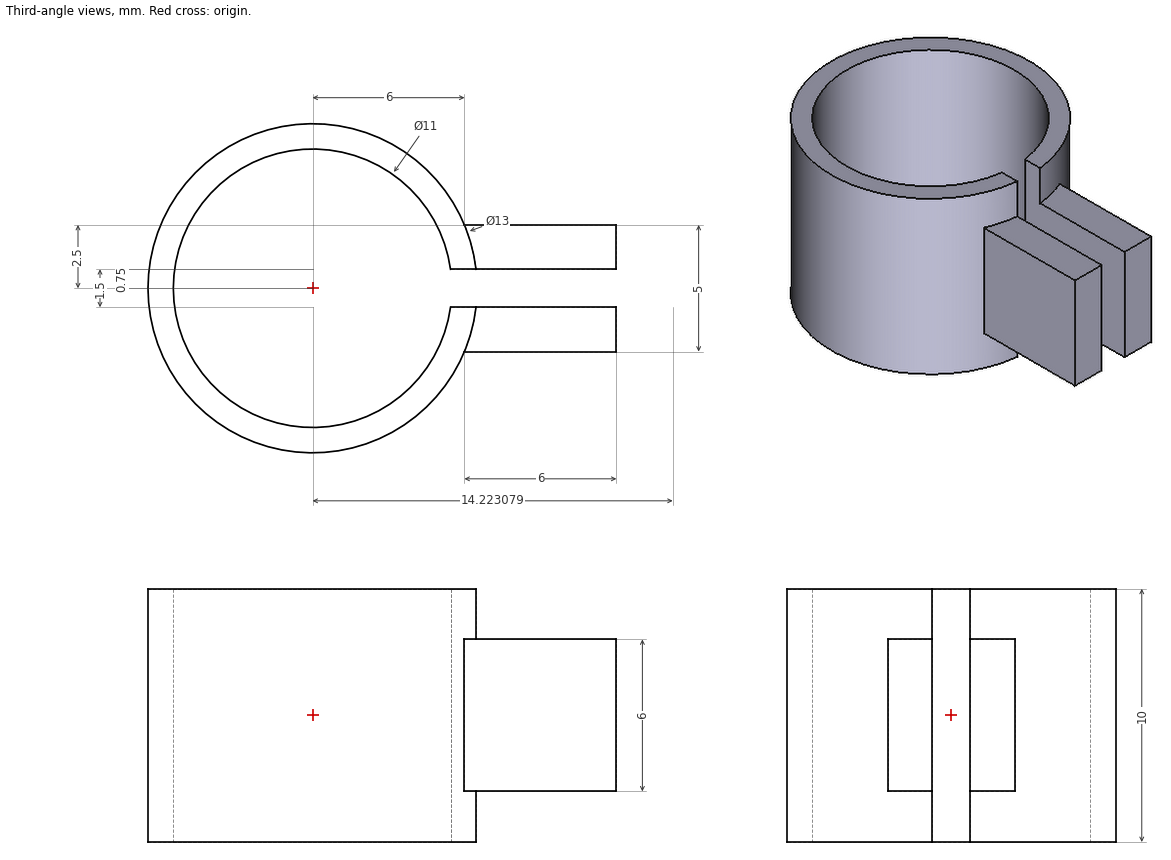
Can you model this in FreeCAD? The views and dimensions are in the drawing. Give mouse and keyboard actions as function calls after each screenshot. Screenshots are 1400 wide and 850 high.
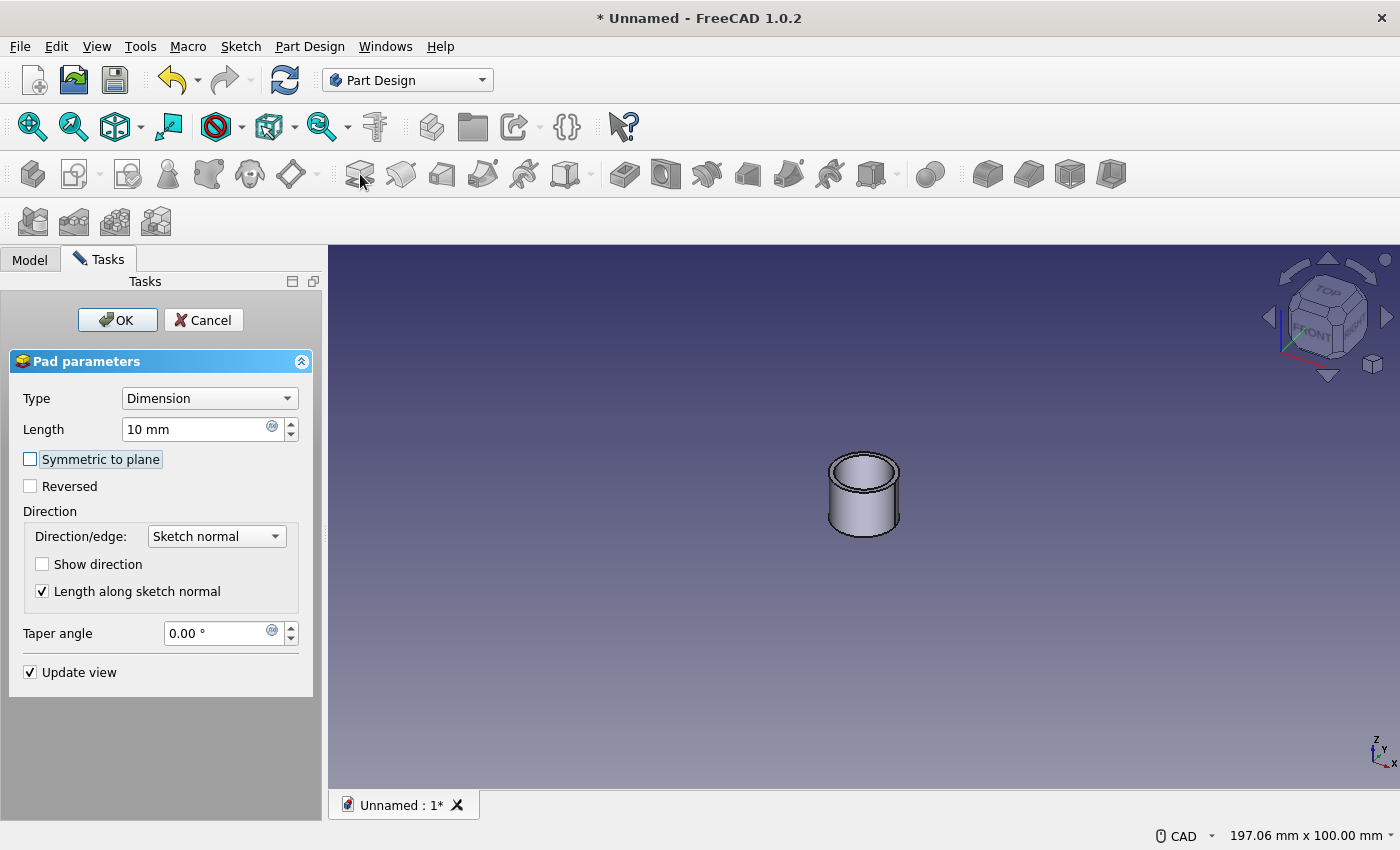
click(31, 459)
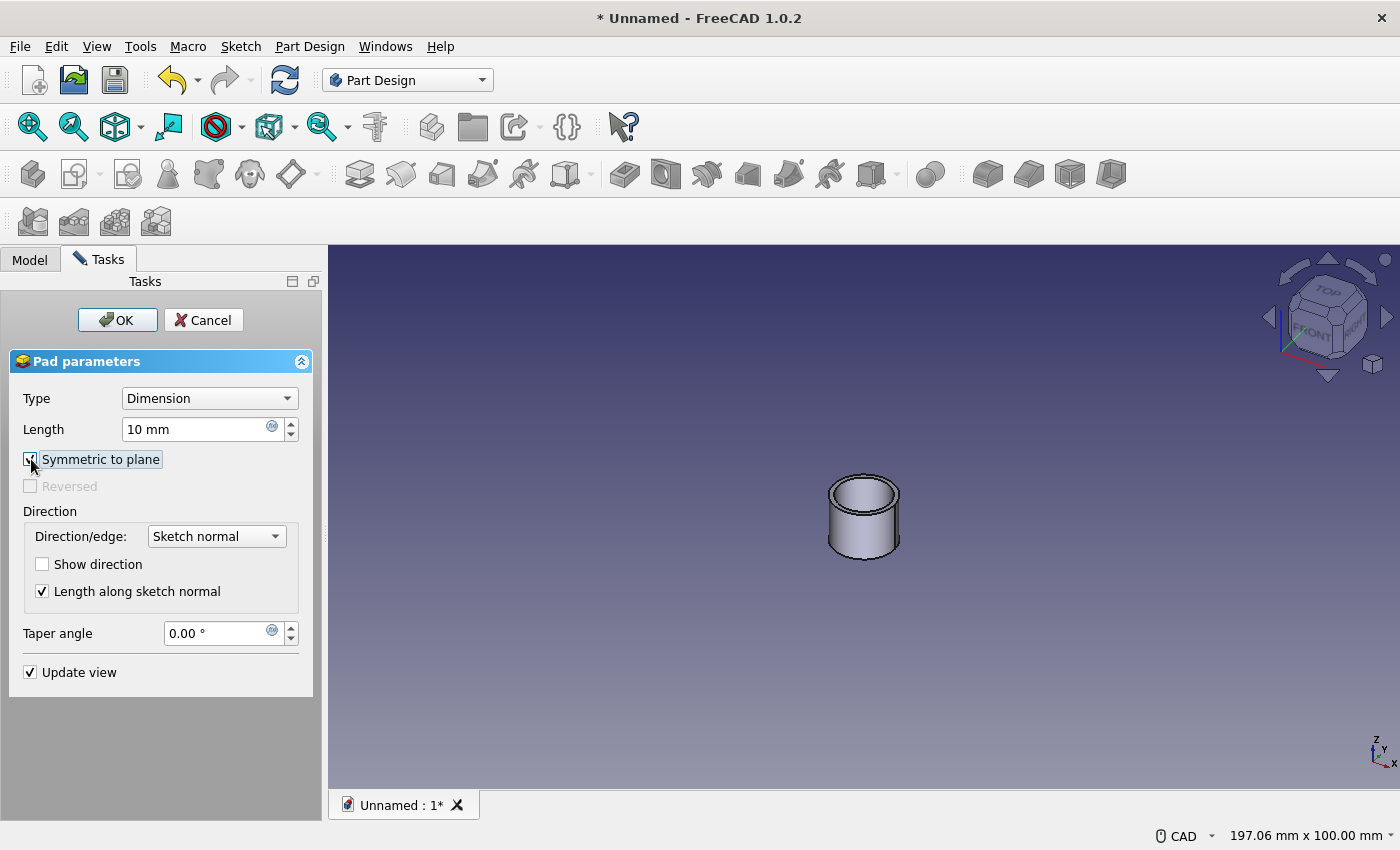
click(118, 320)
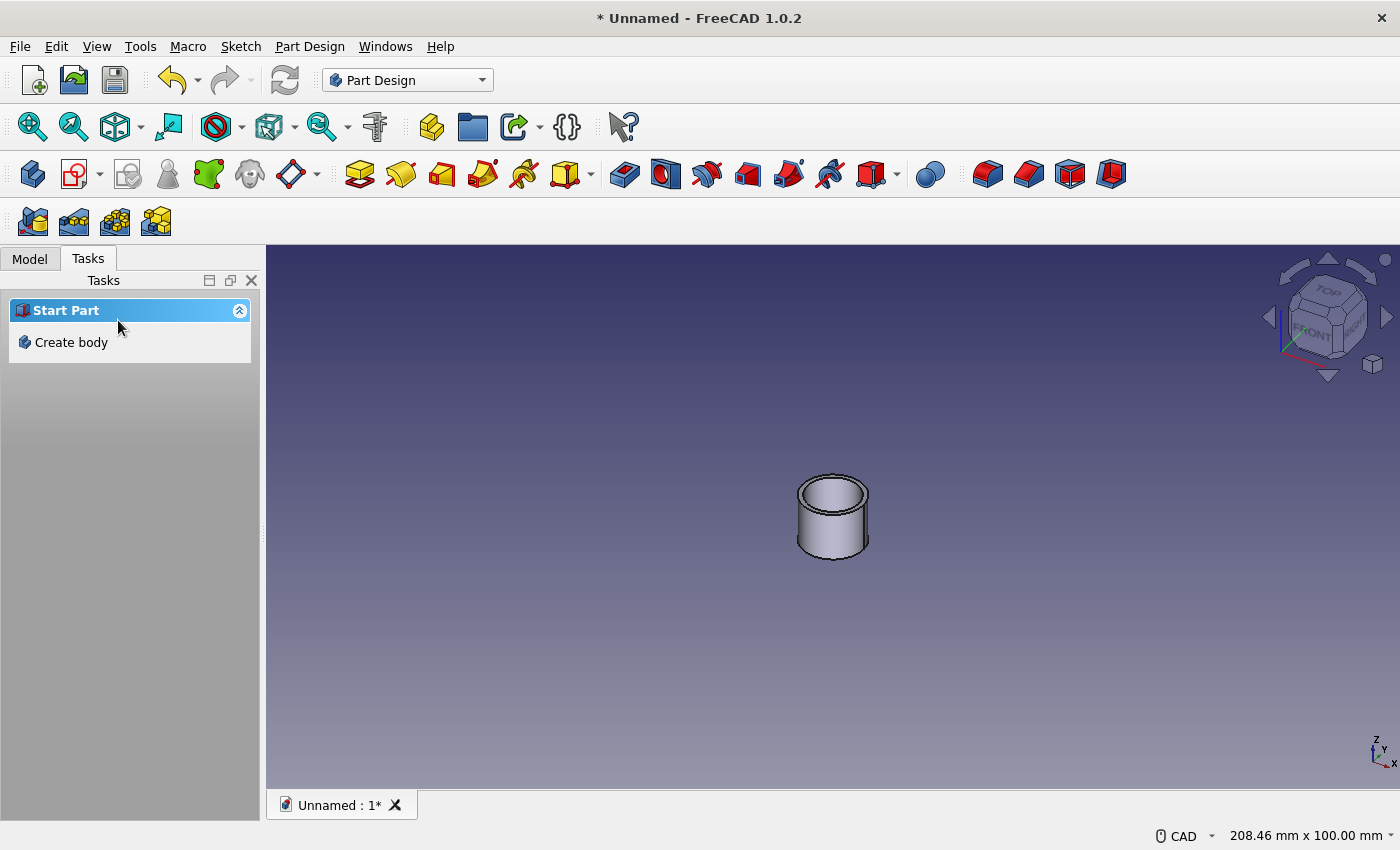
key(v)
key(f)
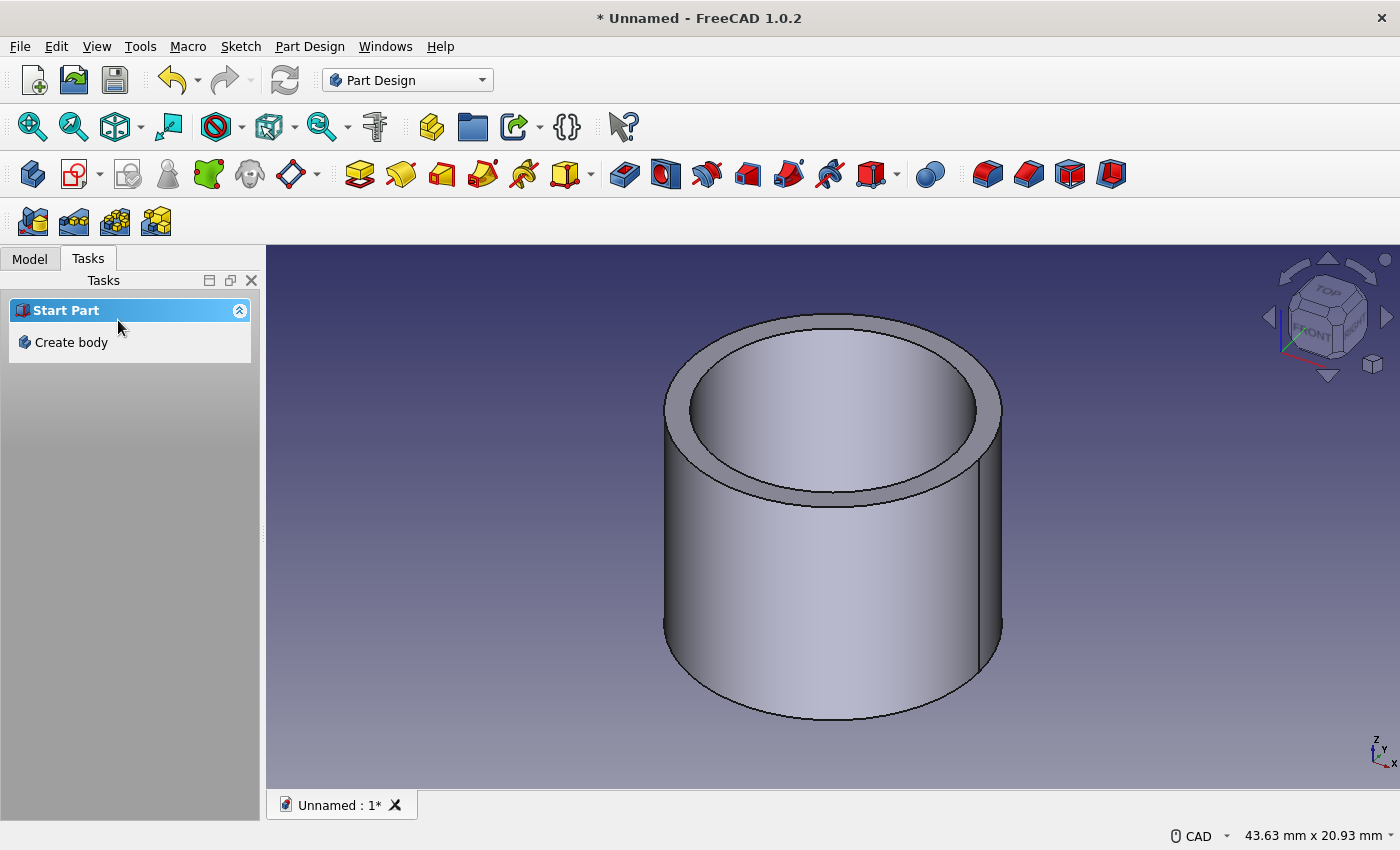
click(74, 174)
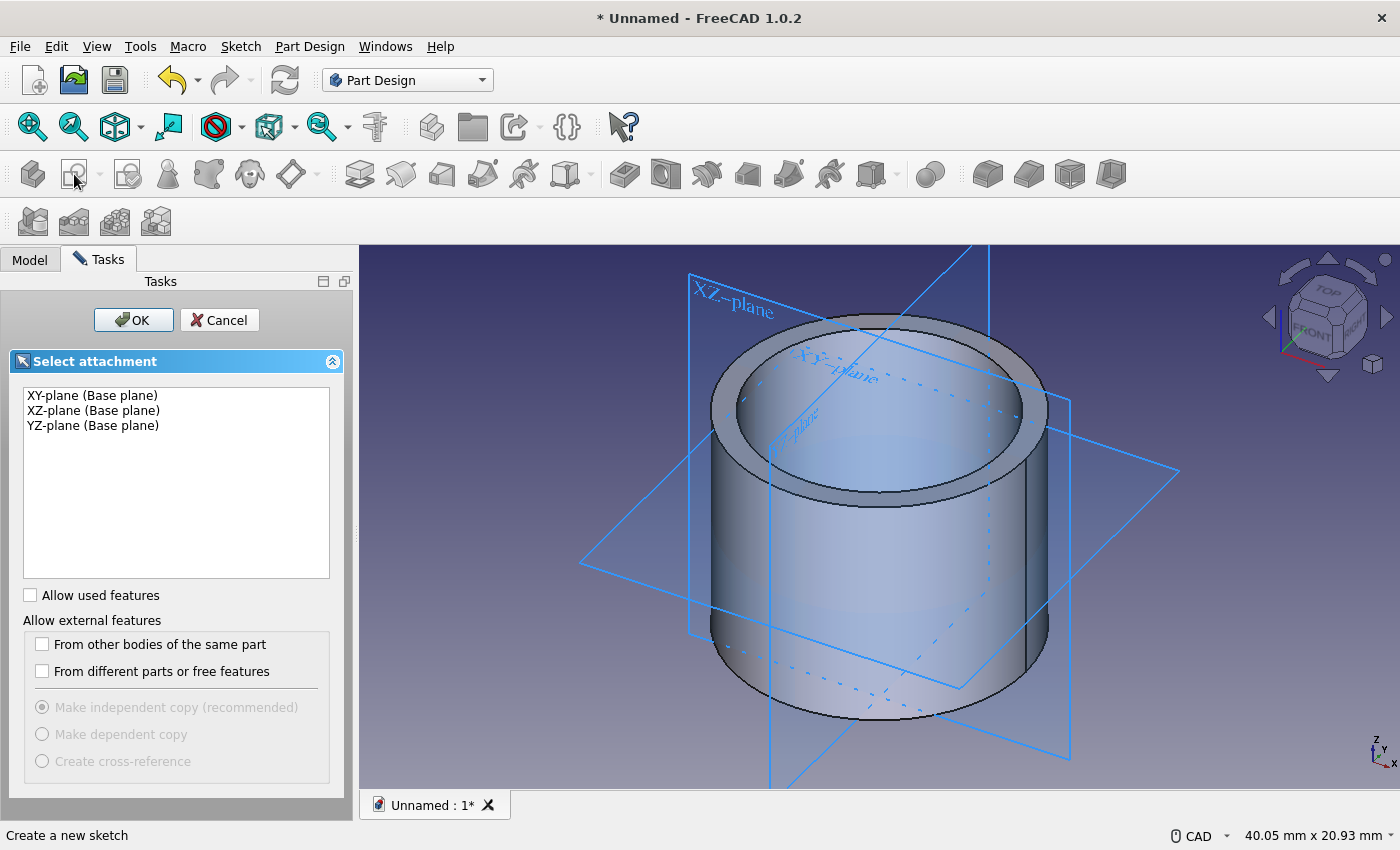
click(84, 396)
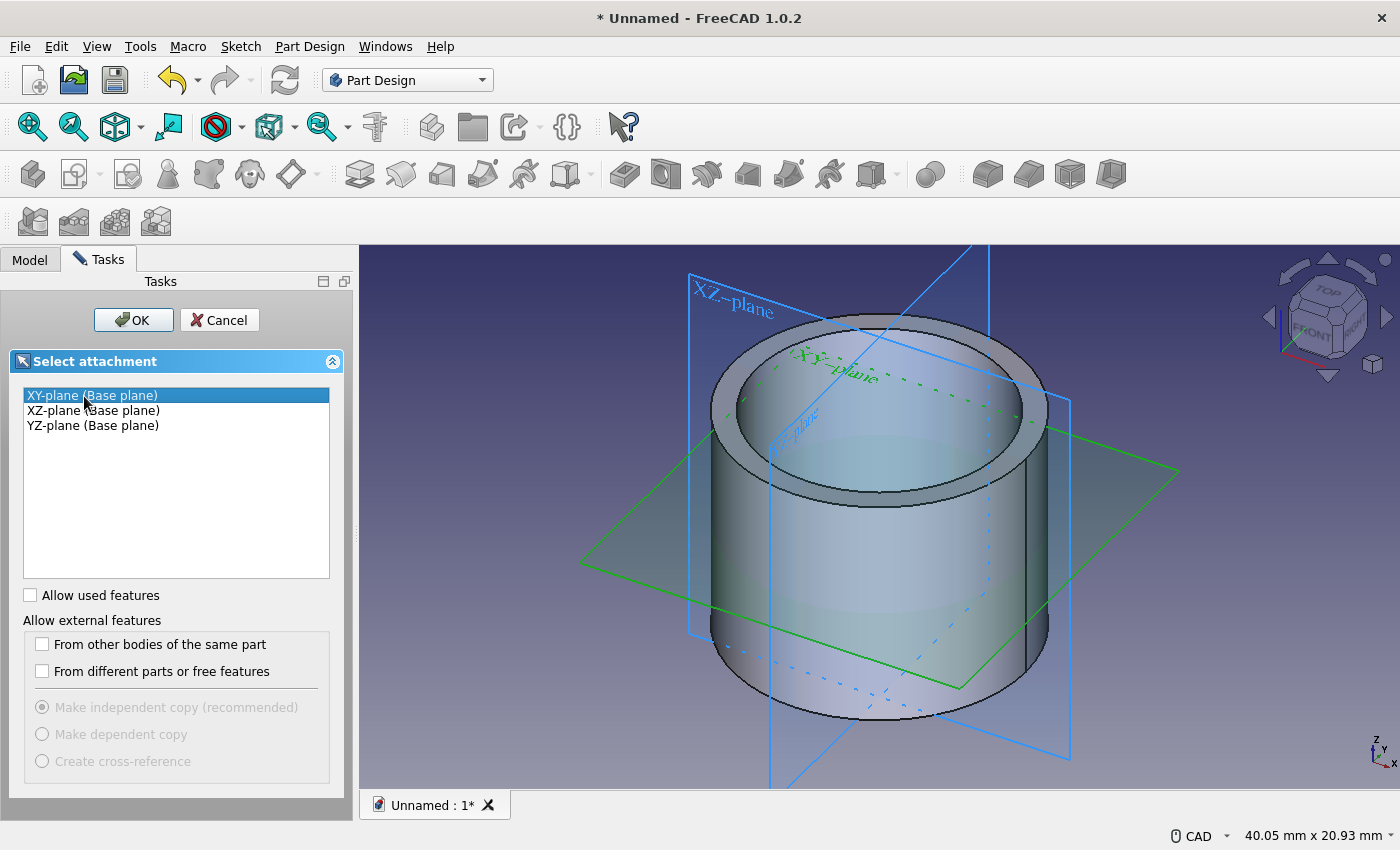
click(134, 320)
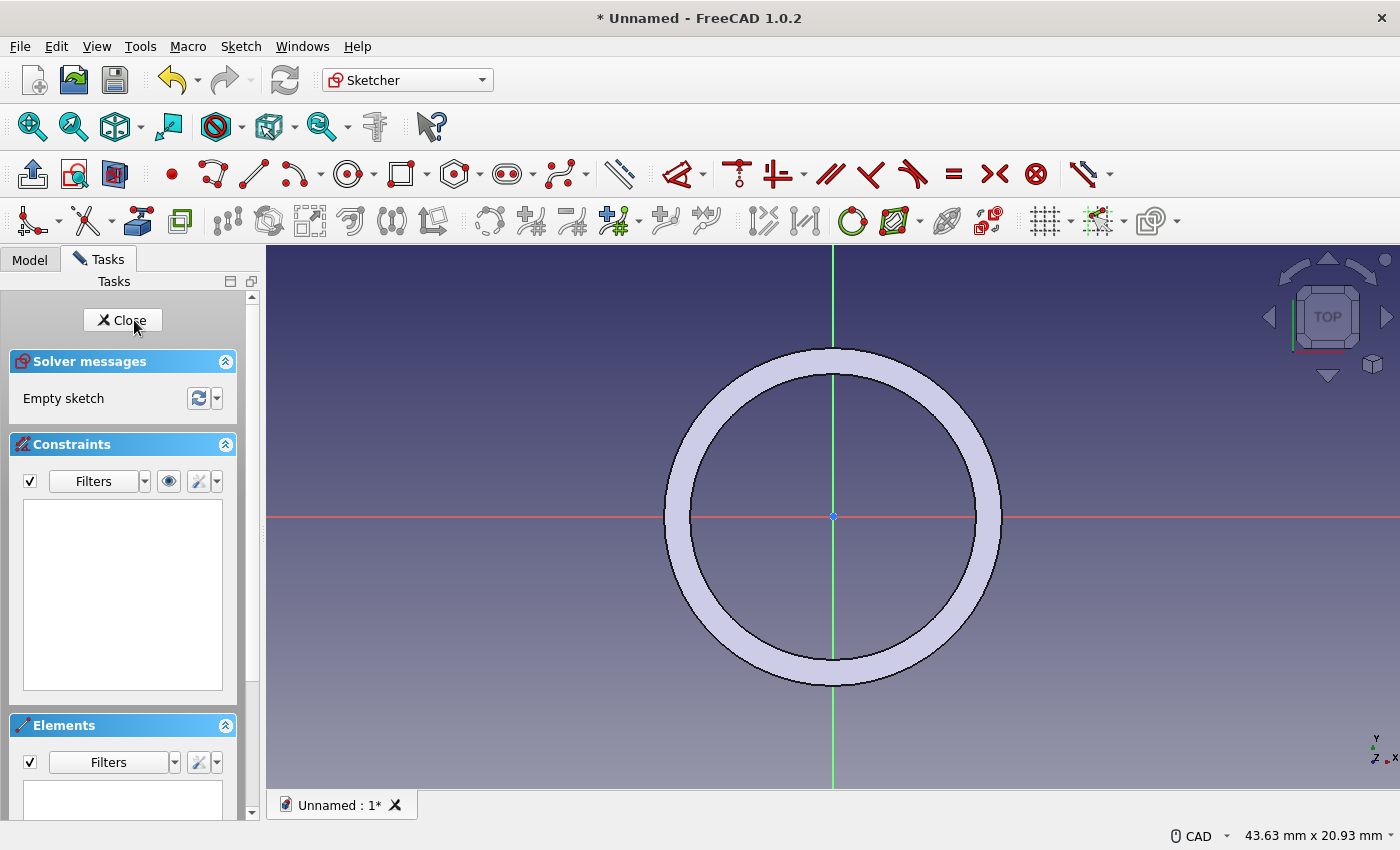
key(q)
key(s)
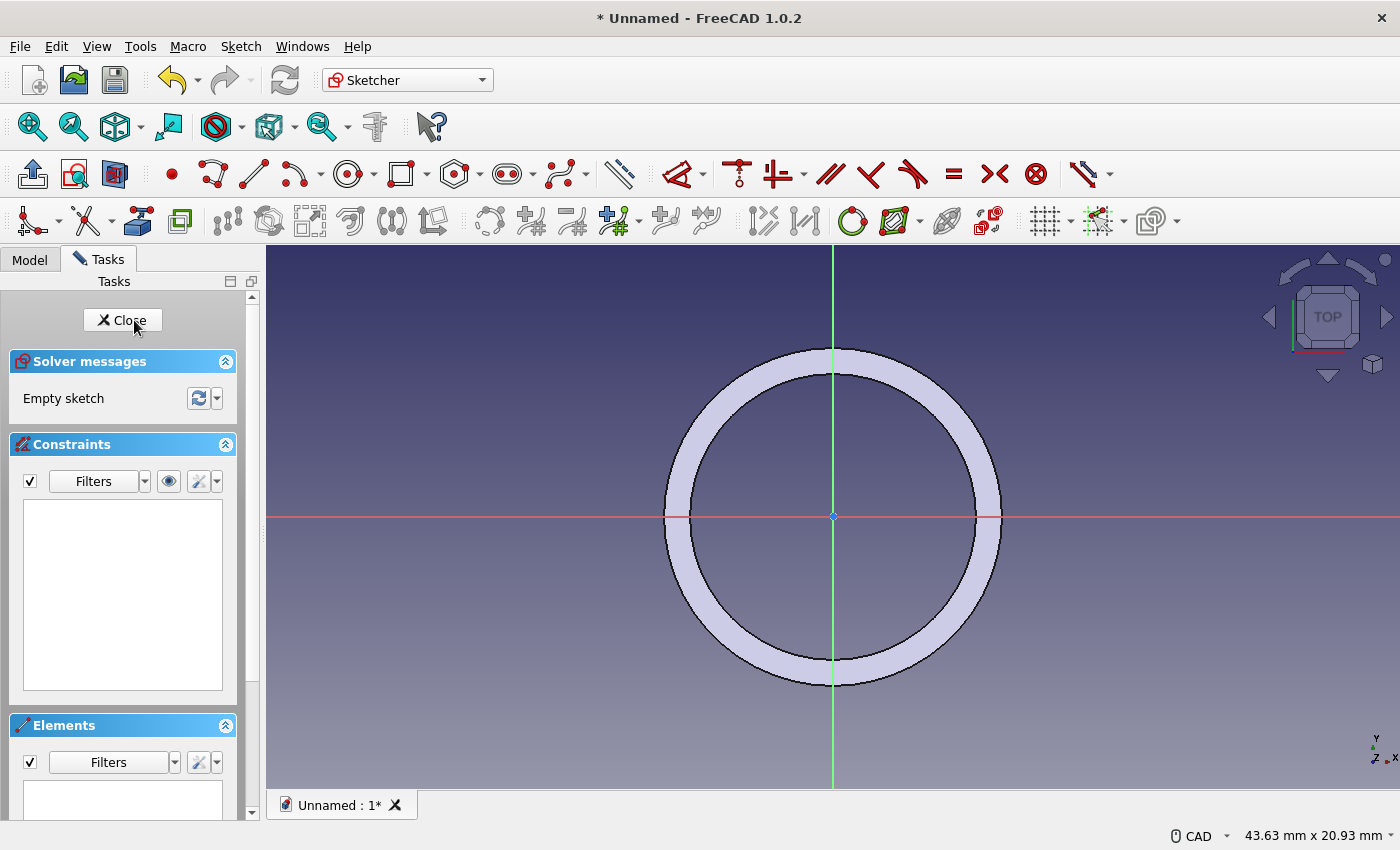
scroll(1172, 517, up, 4)